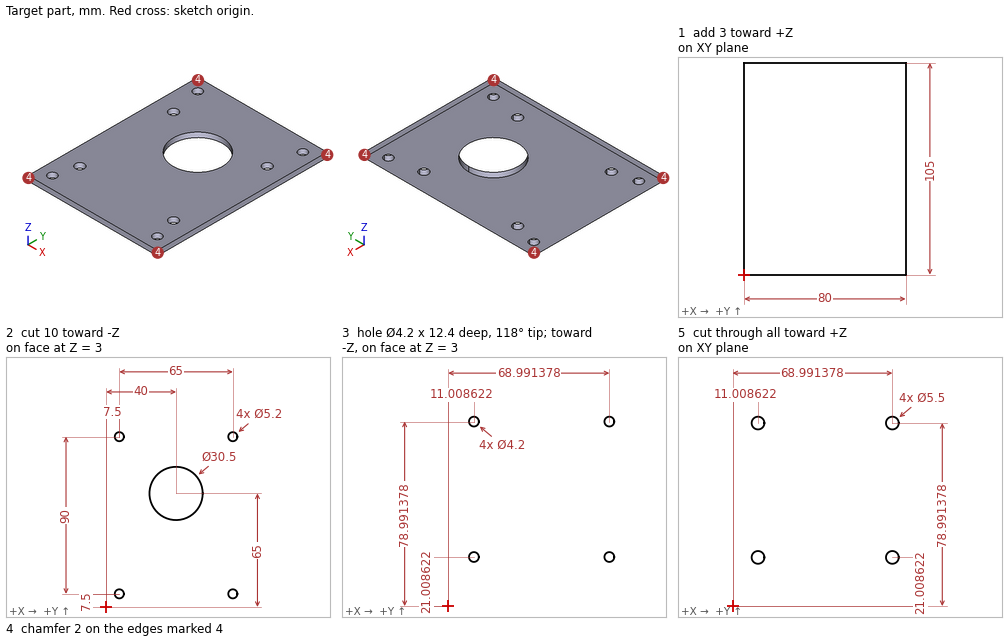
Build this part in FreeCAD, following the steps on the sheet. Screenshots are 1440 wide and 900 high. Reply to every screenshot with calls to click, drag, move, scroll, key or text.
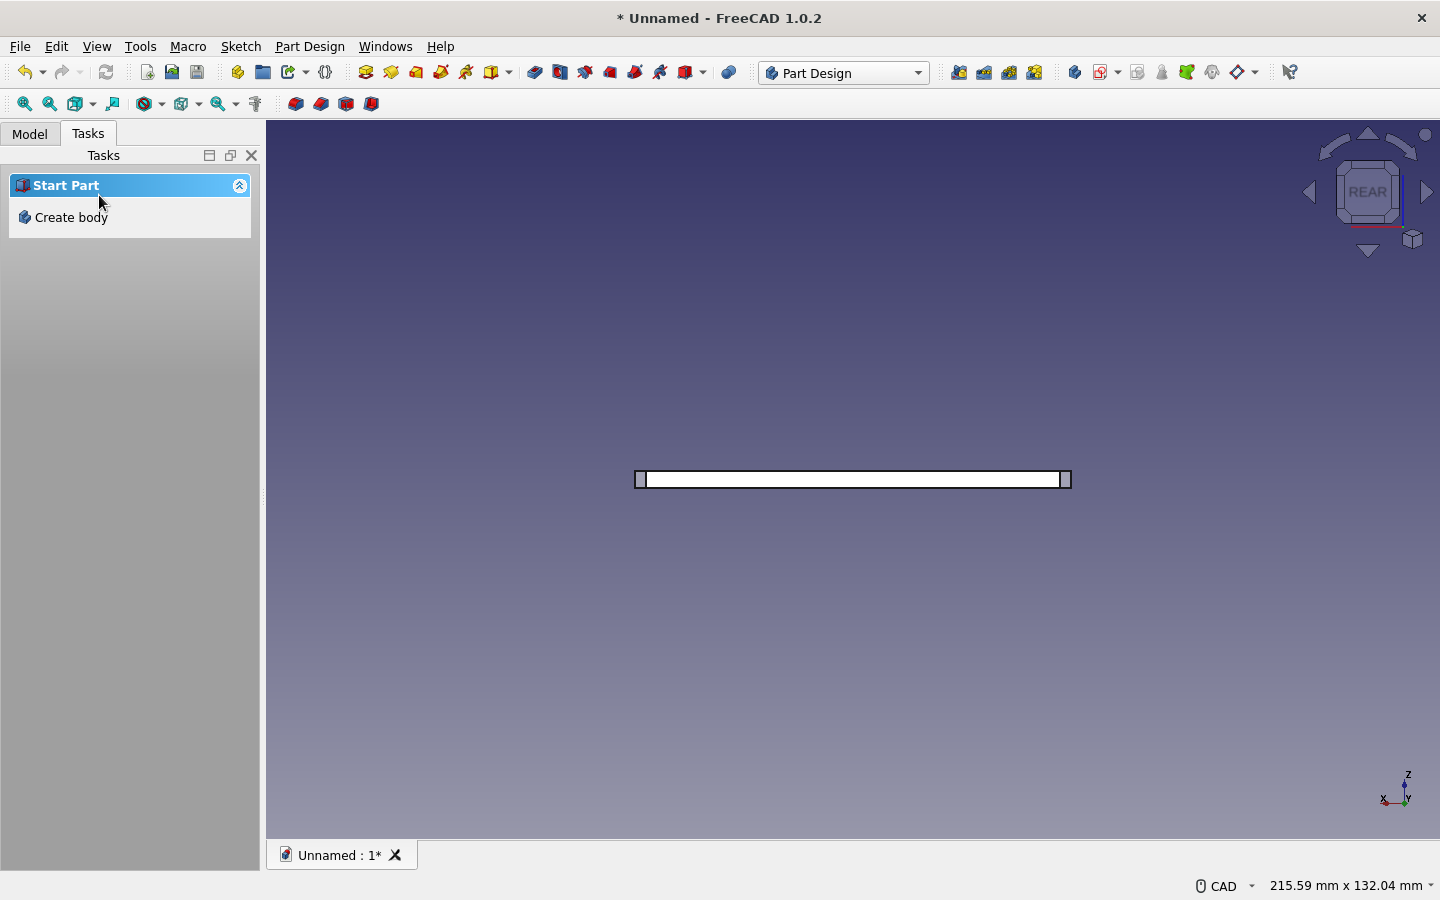
click(25, 104)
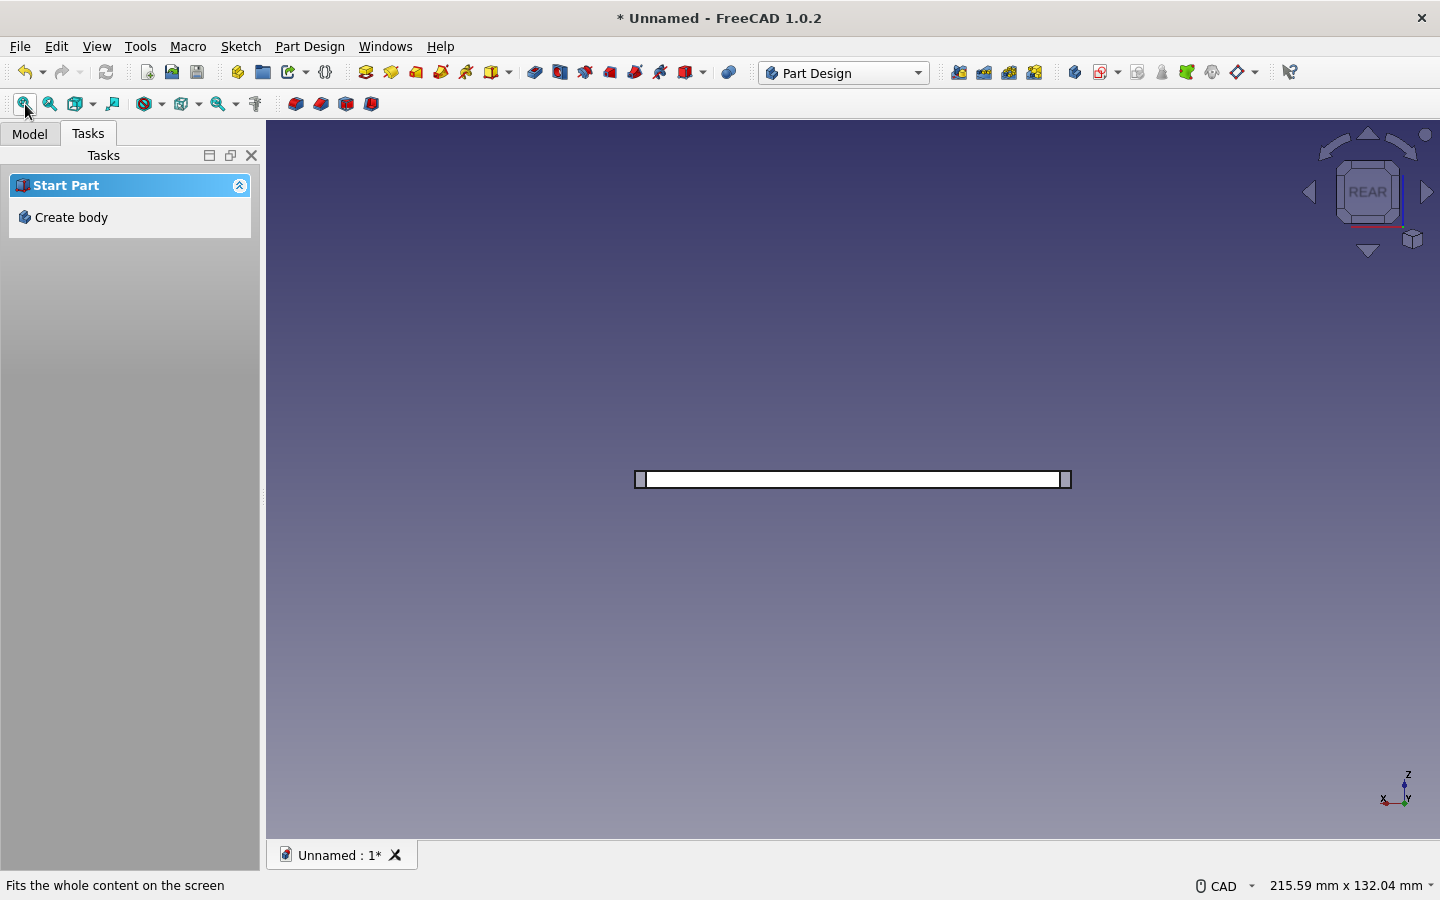
click(1100, 72)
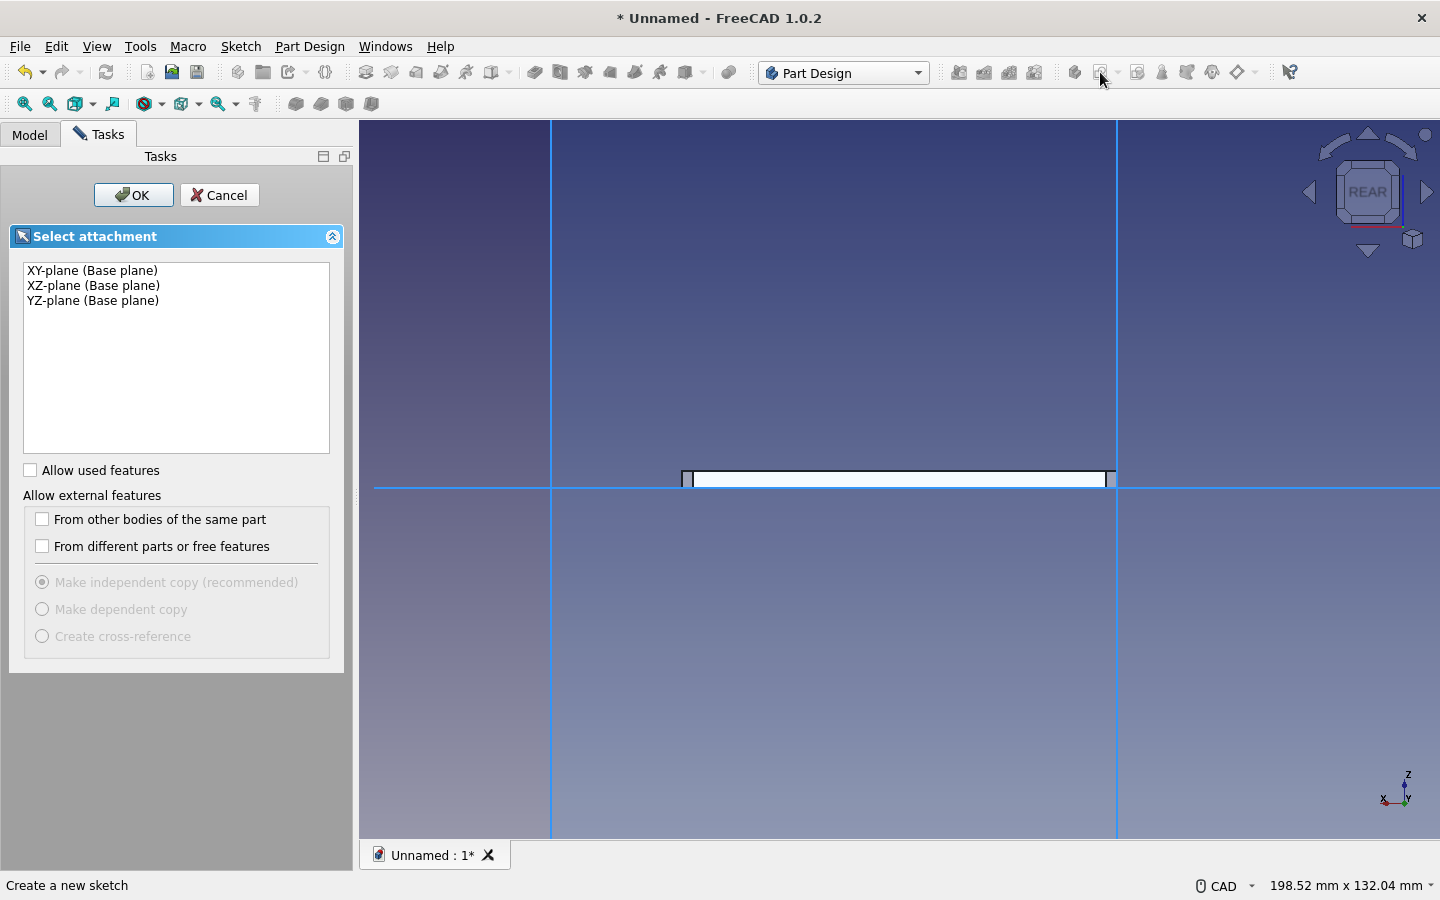
click(84, 270)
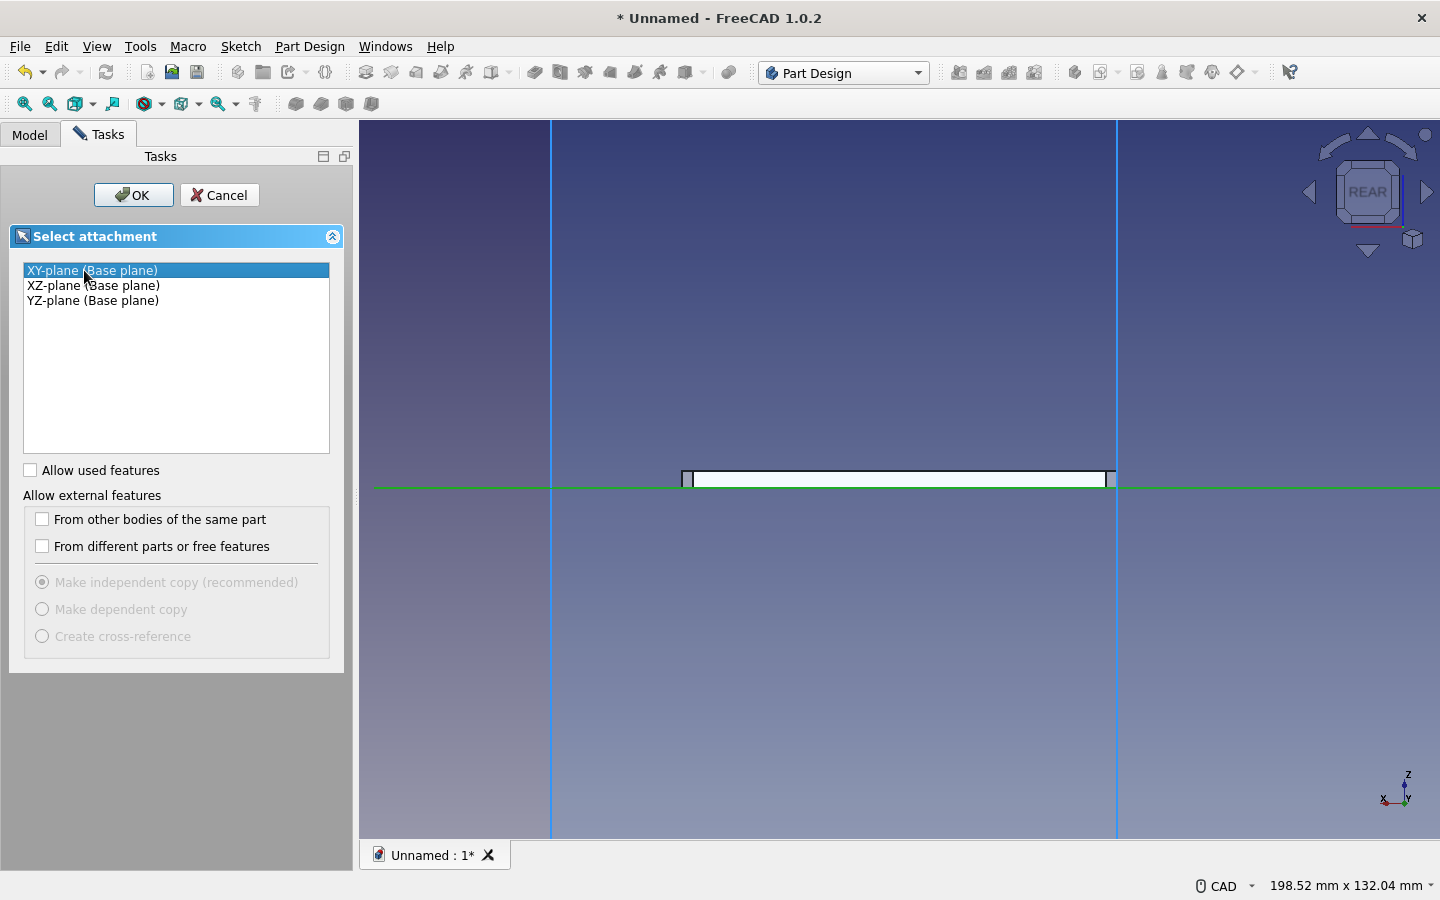
click(134, 195)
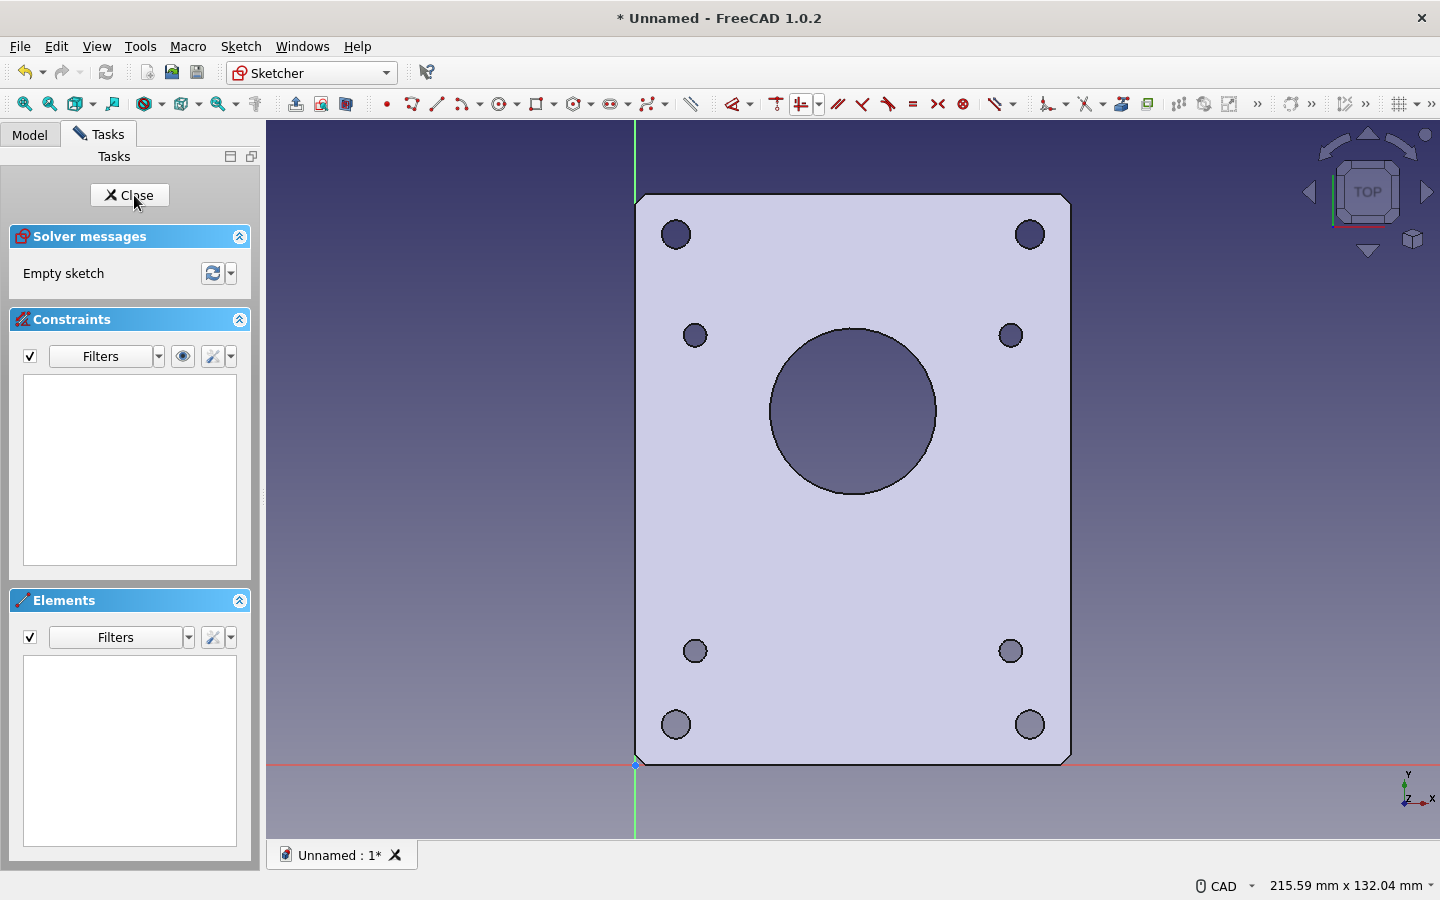
click(346, 104)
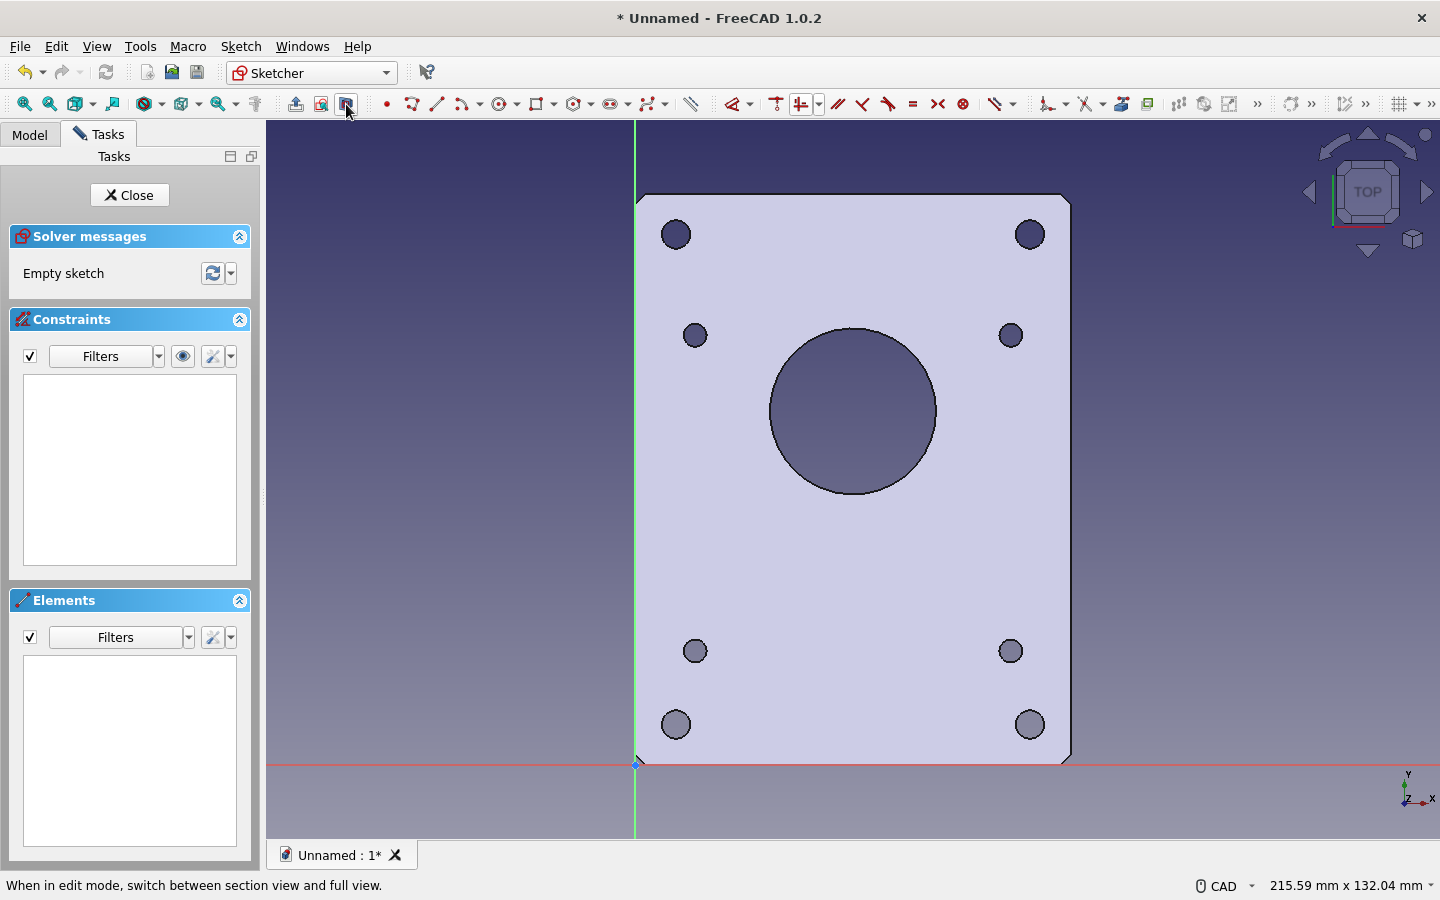
click(498, 104)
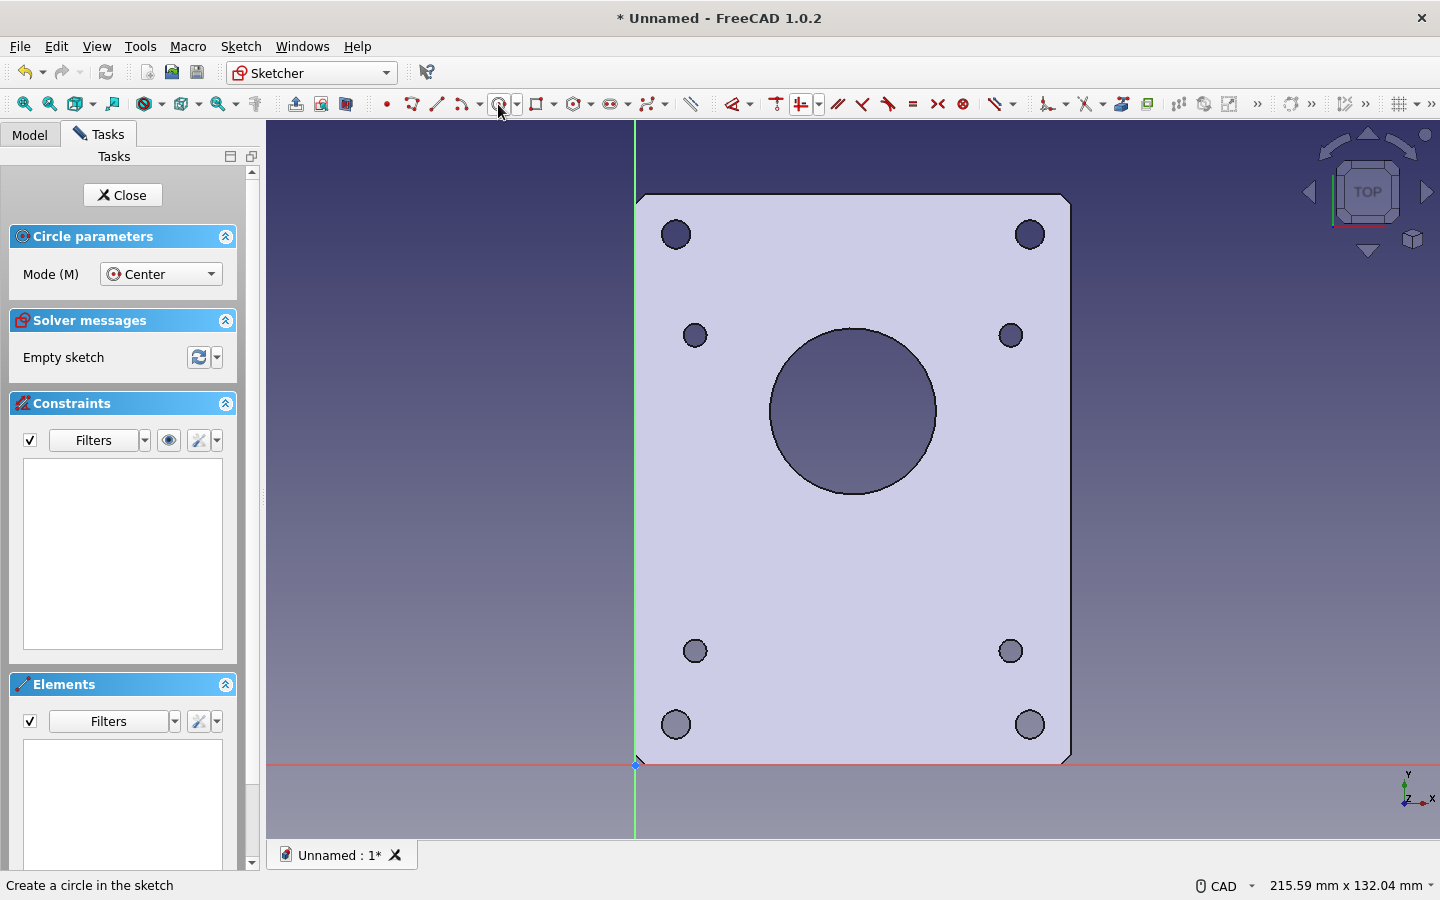
scroll(1011, 335, up, 3)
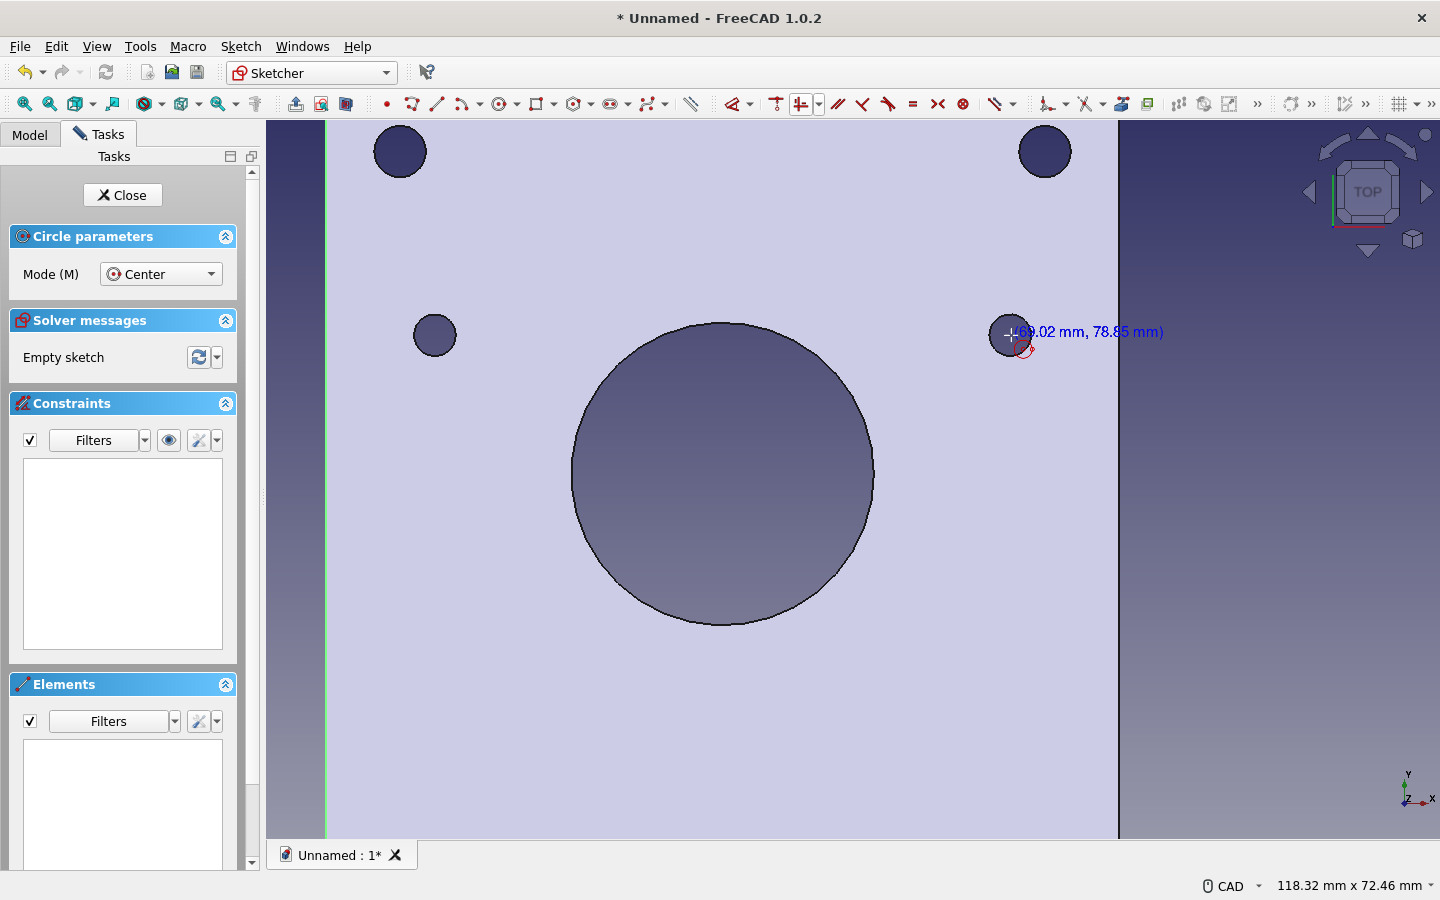
click(1010, 335)
click(1030, 316)